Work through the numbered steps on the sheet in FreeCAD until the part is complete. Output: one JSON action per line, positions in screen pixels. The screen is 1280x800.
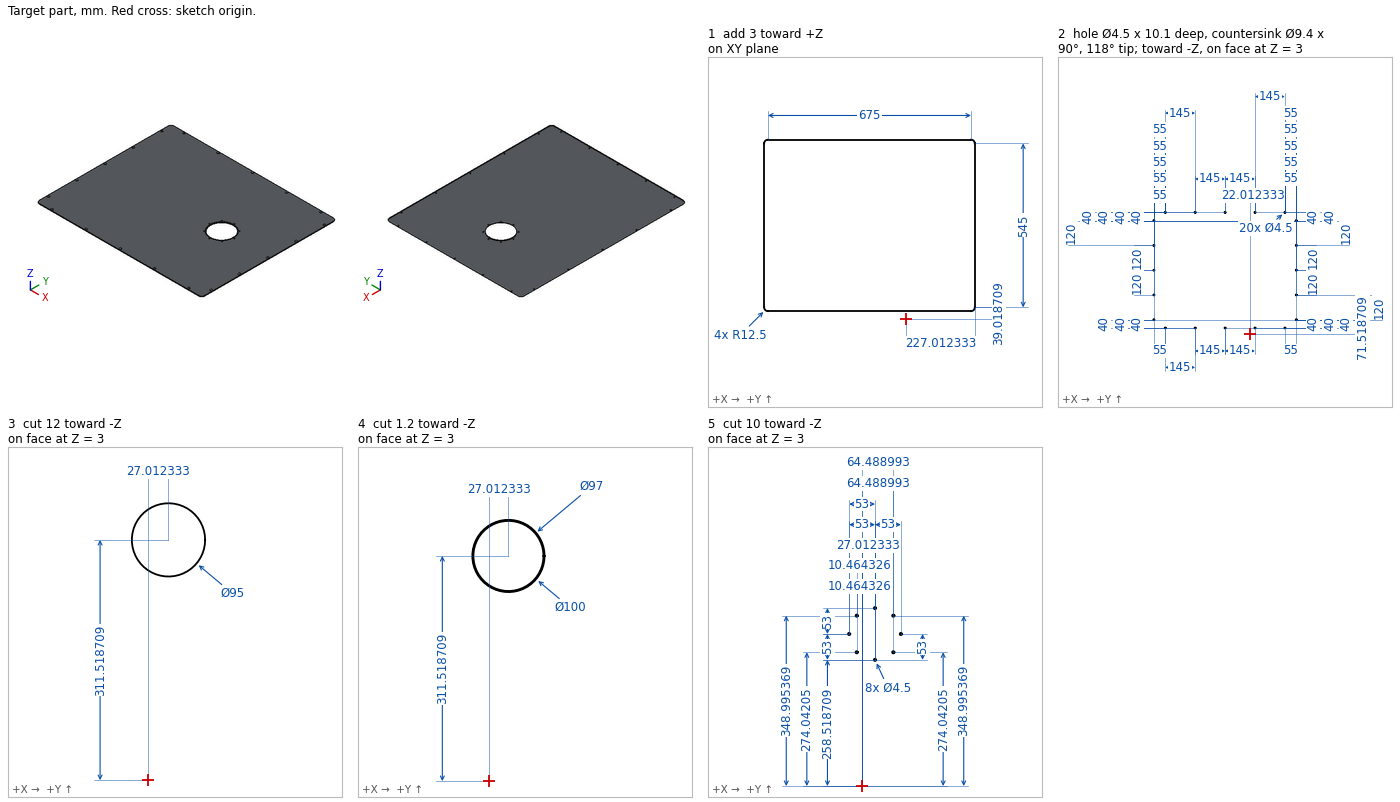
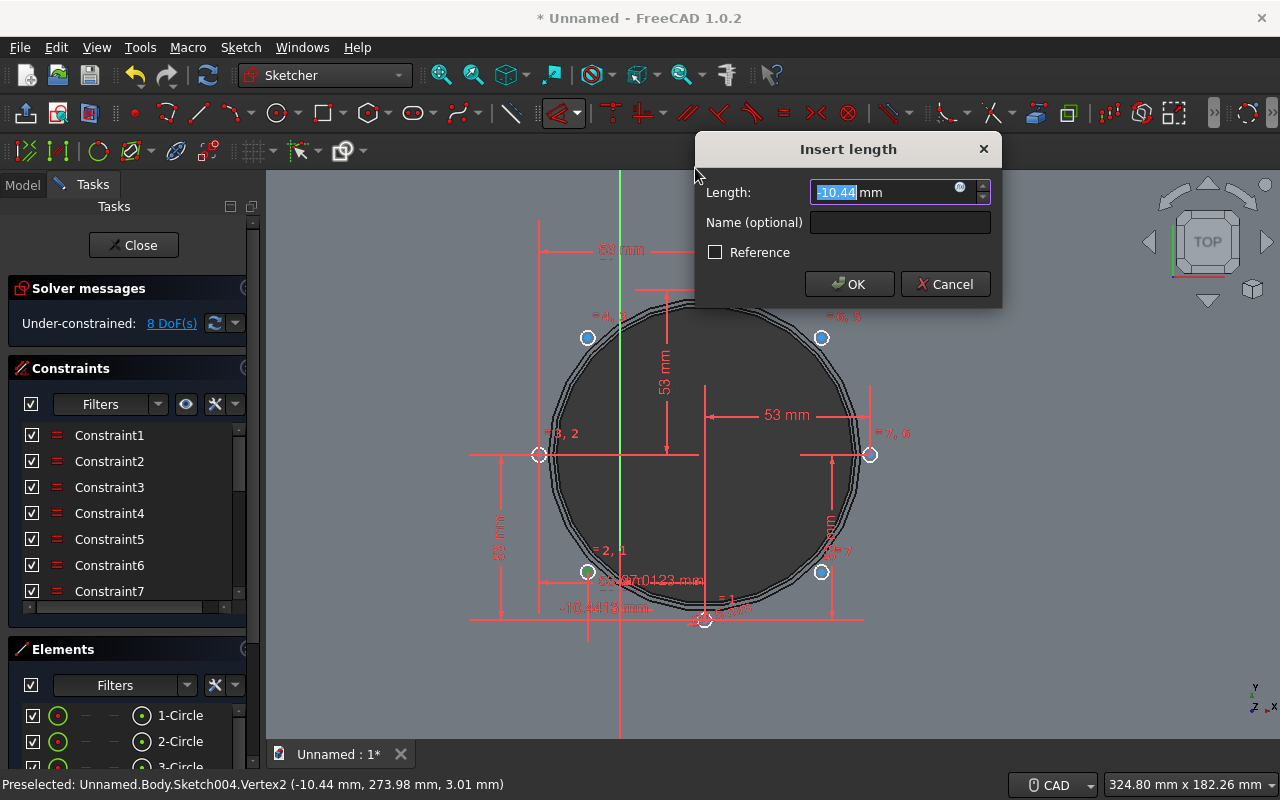
{"action": "type", "text": "-10.464326"}
{"action": "key", "text": "Return"}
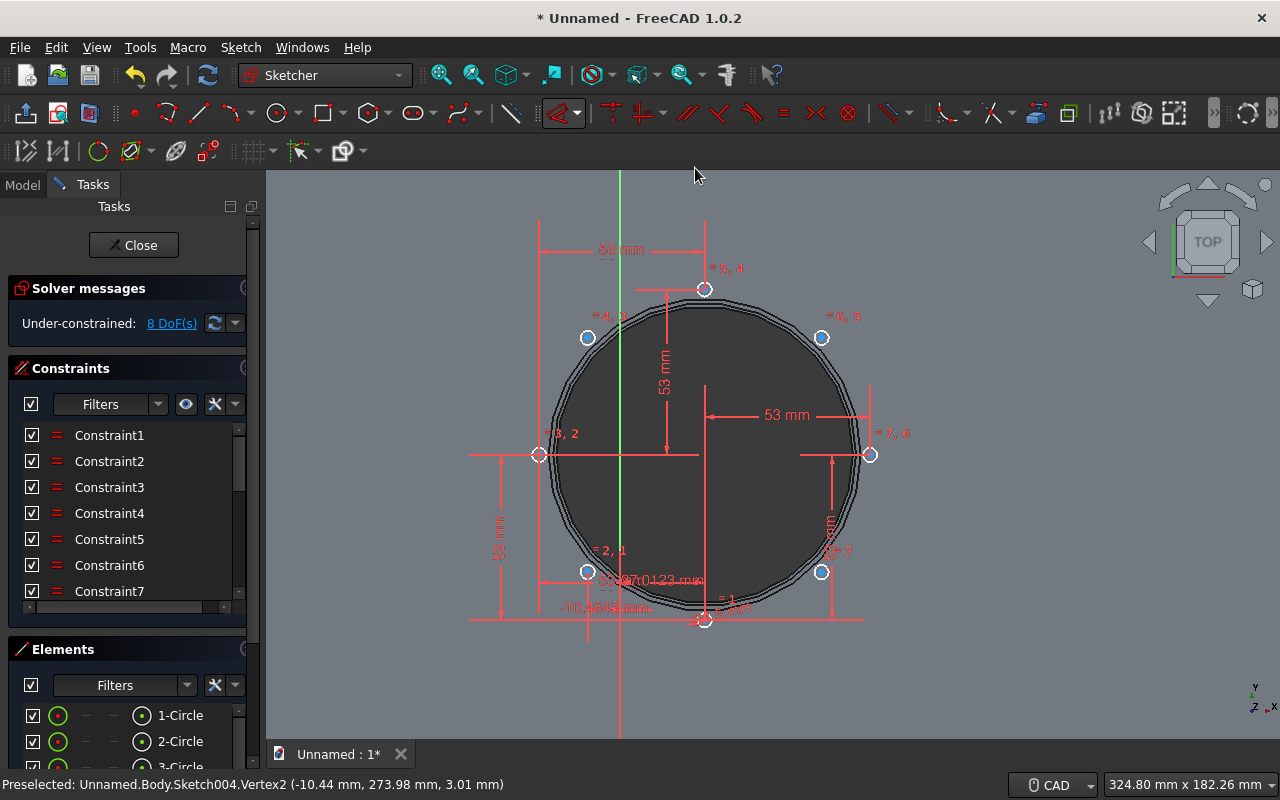
{"action": "left_click", "coordinate": [588, 572]}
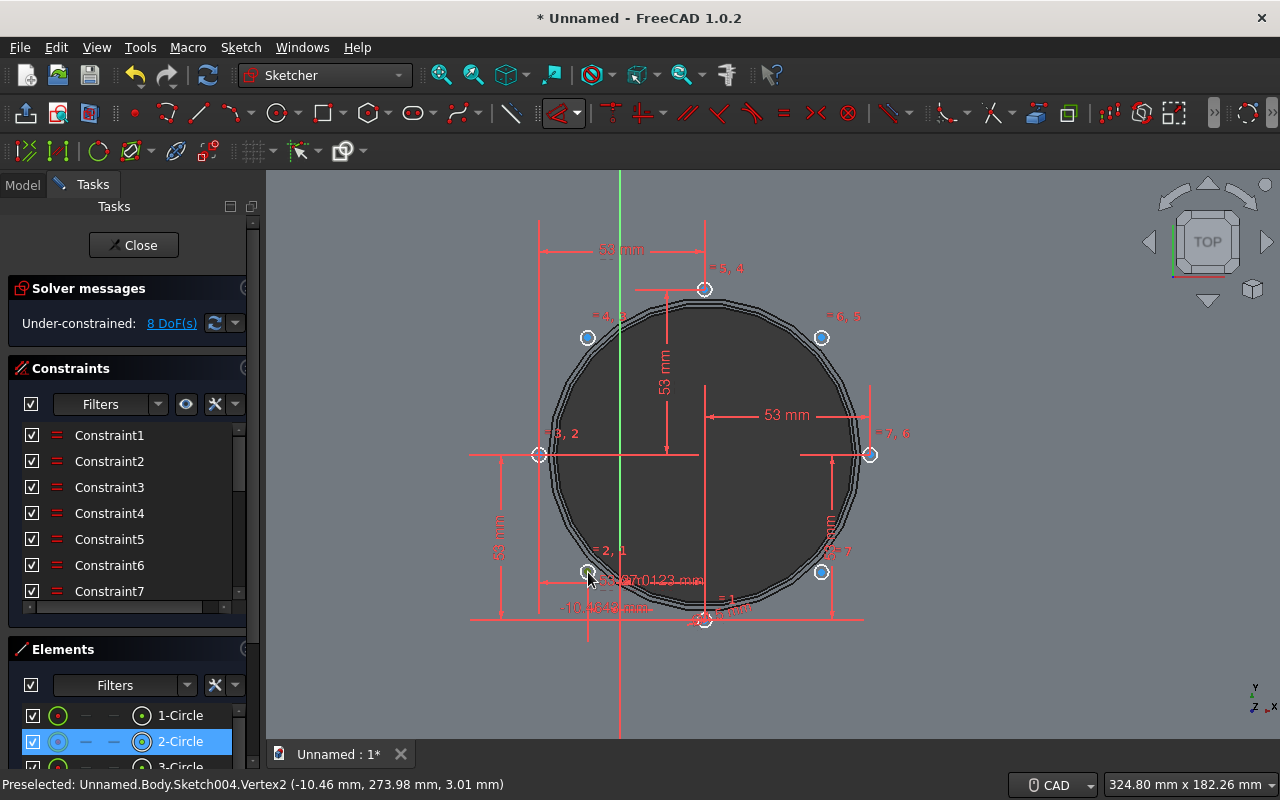
{"action": "left_click", "coordinate": [580, 114]}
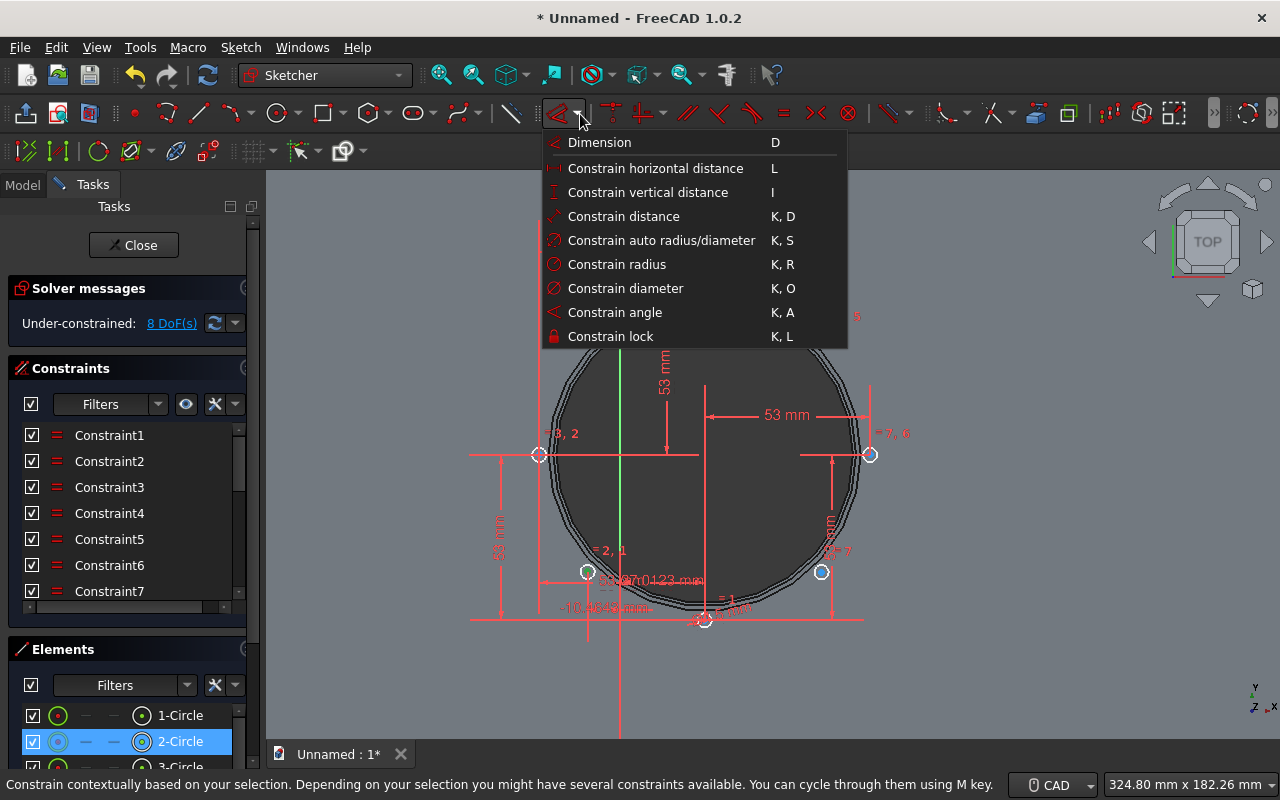
{"action": "left_click", "coordinate": [695, 192]}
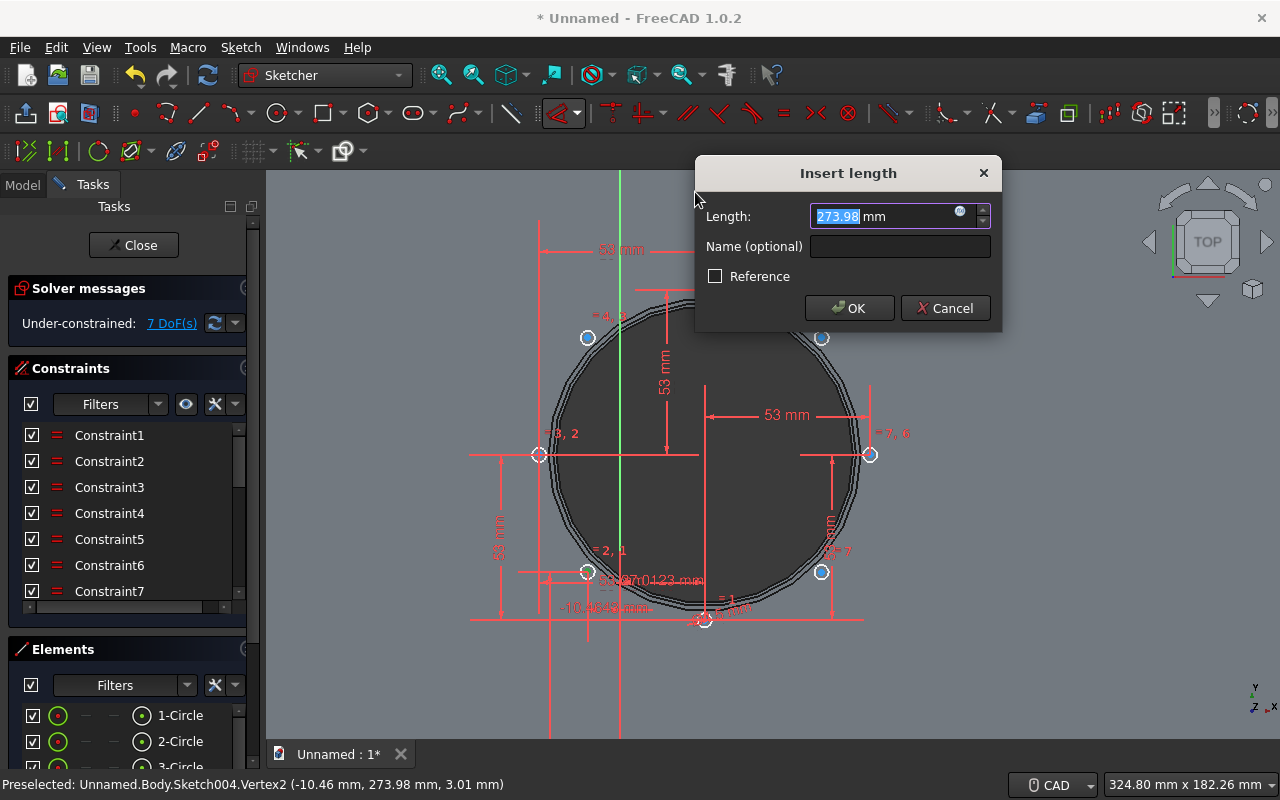
{"action": "type", "text": "274.04205"}
{"action": "key", "text": "Return"}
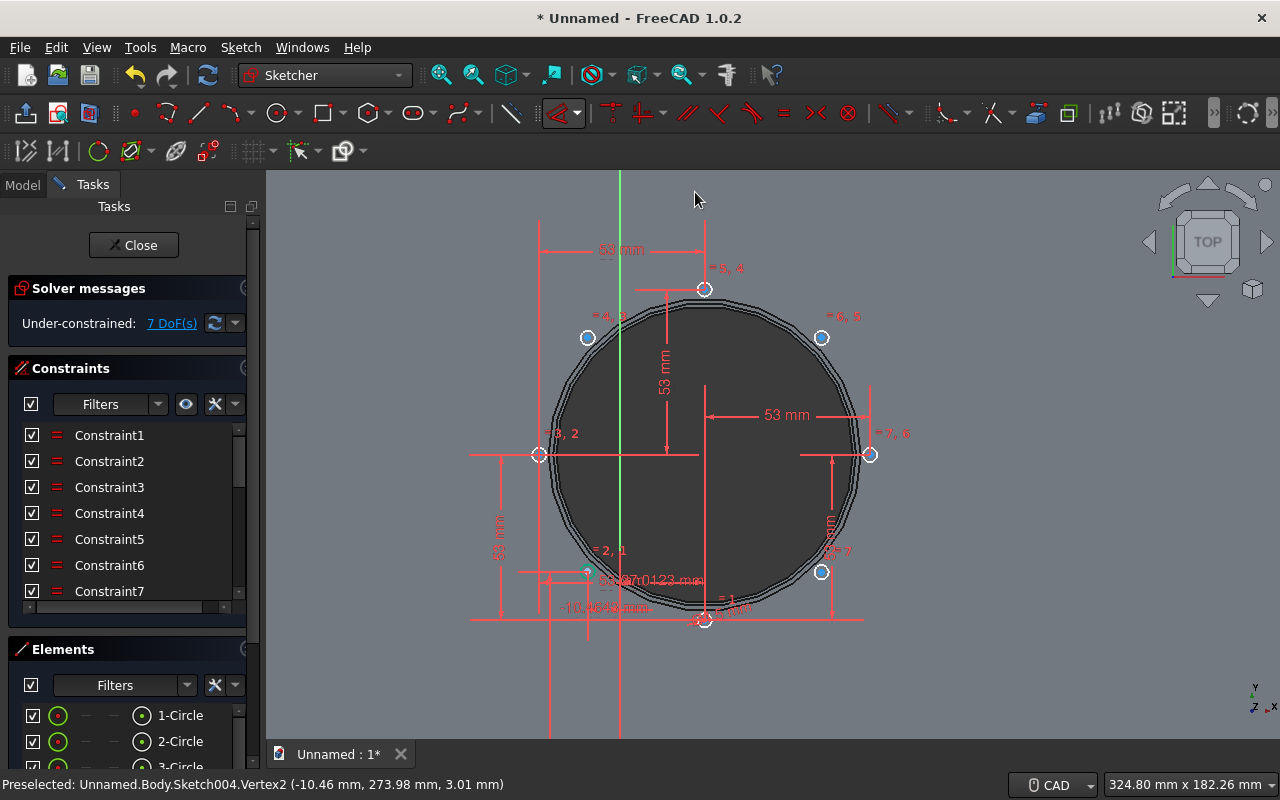
{"action": "left_click", "coordinate": [588, 338]}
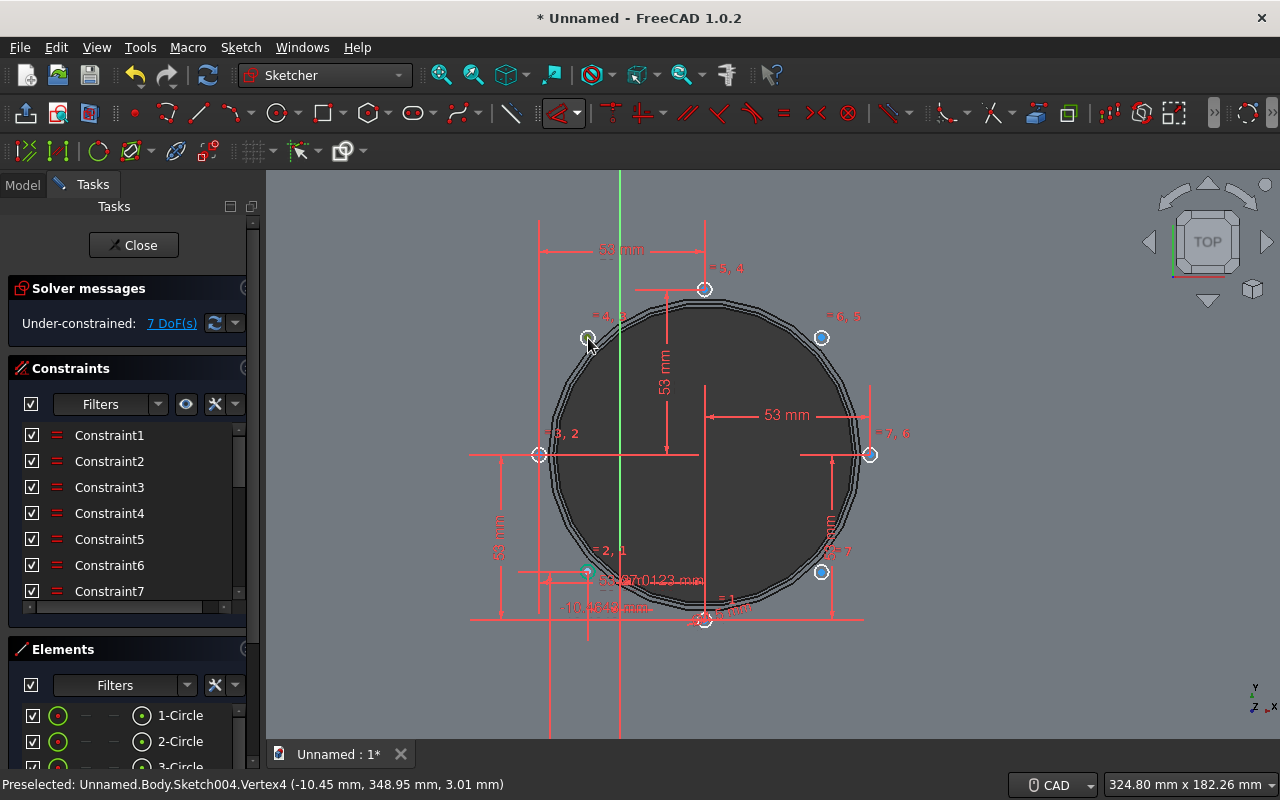
{"action": "left_click", "coordinate": [580, 114]}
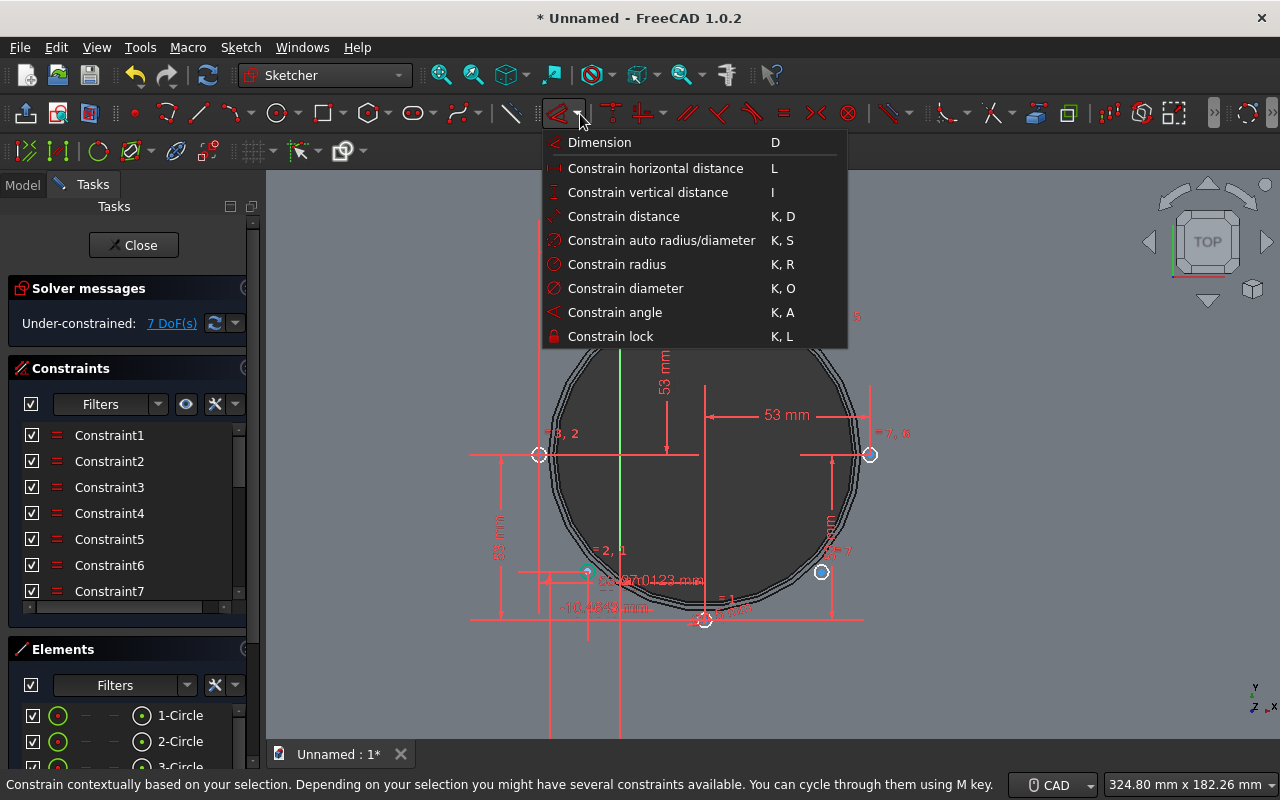
{"action": "left_click", "coordinate": [695, 168]}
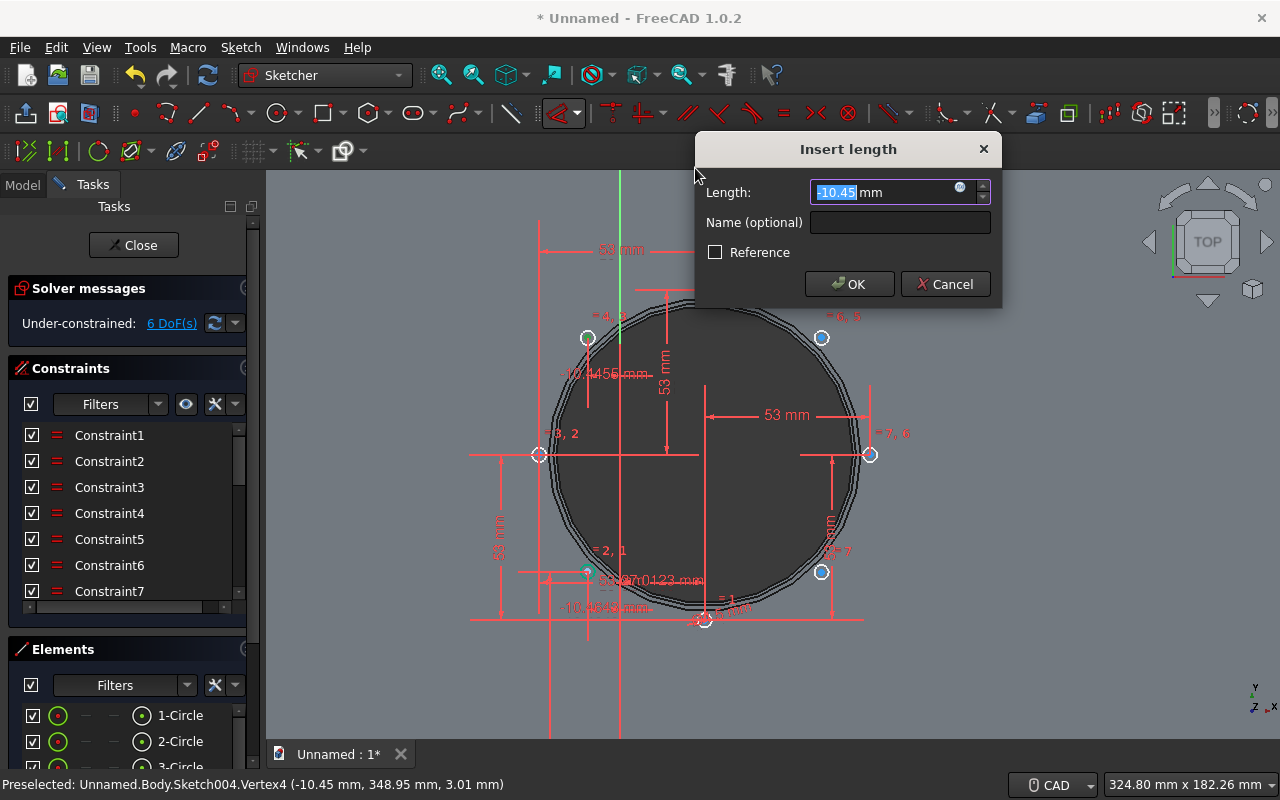
{"action": "type", "text": "-10.464326"}
{"action": "key", "text": "Return"}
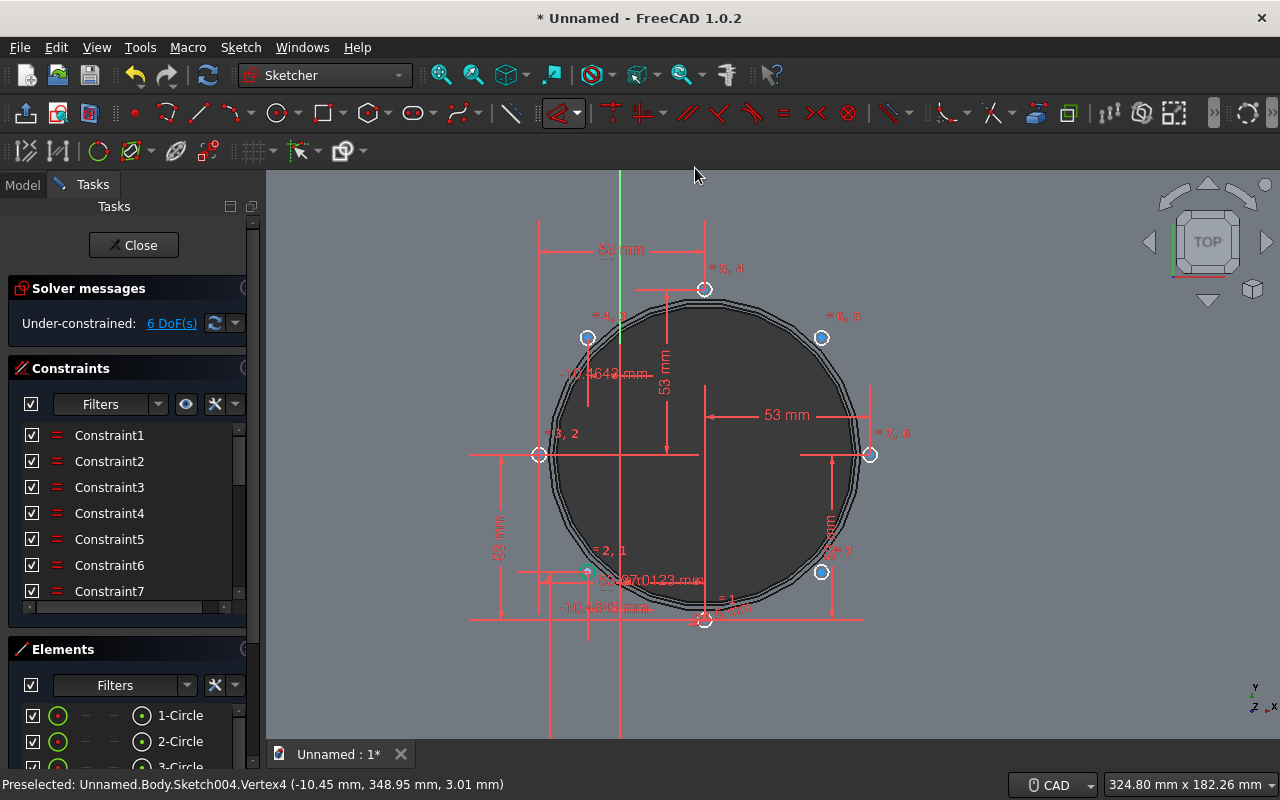
{"action": "left_click", "coordinate": [822, 338]}